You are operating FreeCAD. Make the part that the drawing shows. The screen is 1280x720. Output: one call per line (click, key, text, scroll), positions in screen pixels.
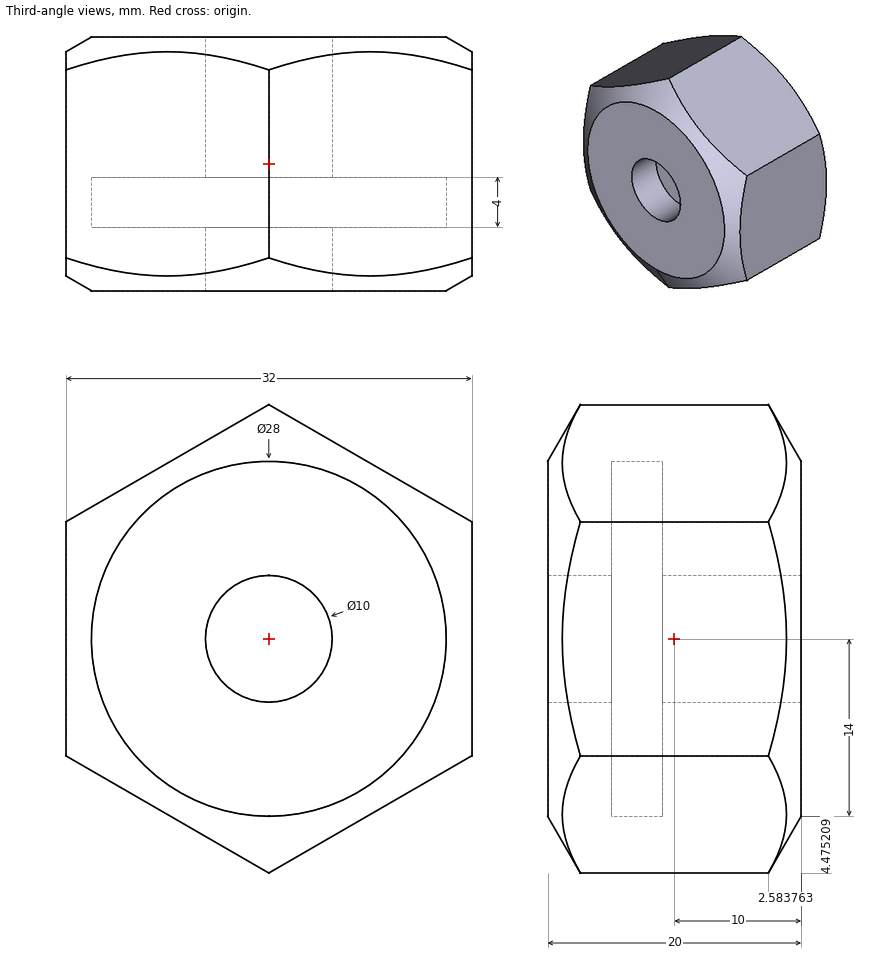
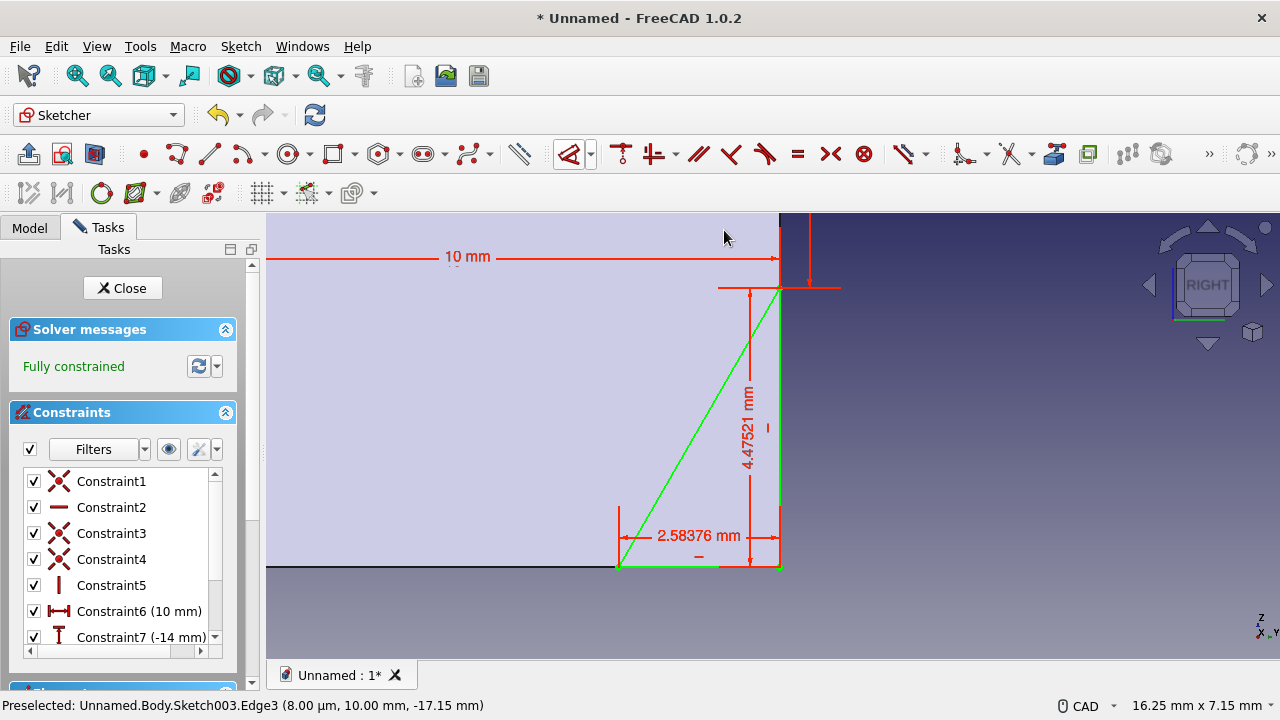
click(123, 288)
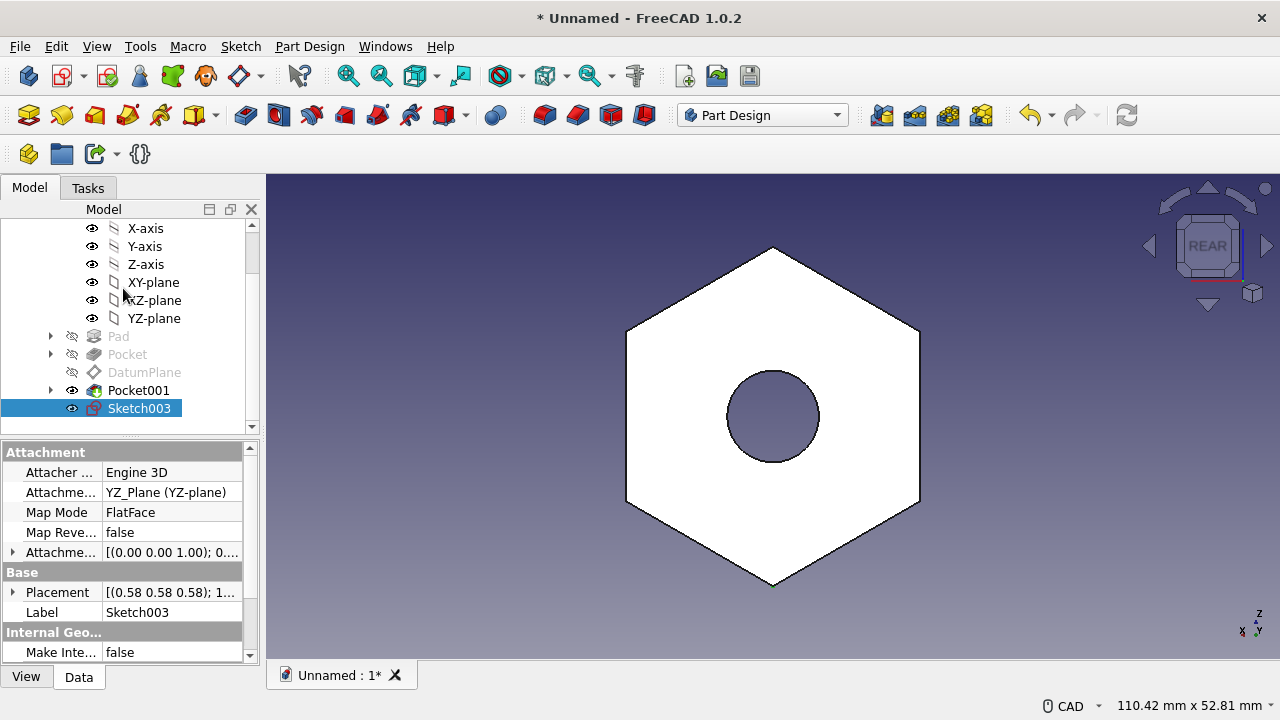
click(312, 116)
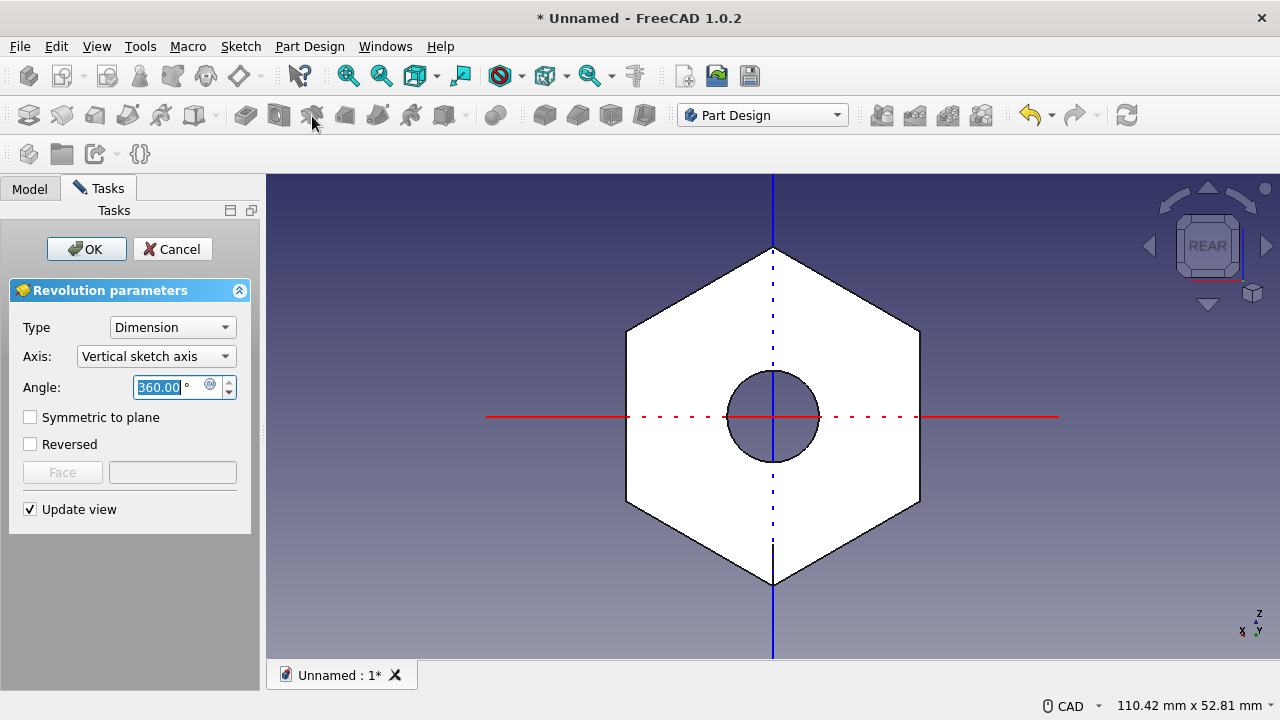
click(157, 356)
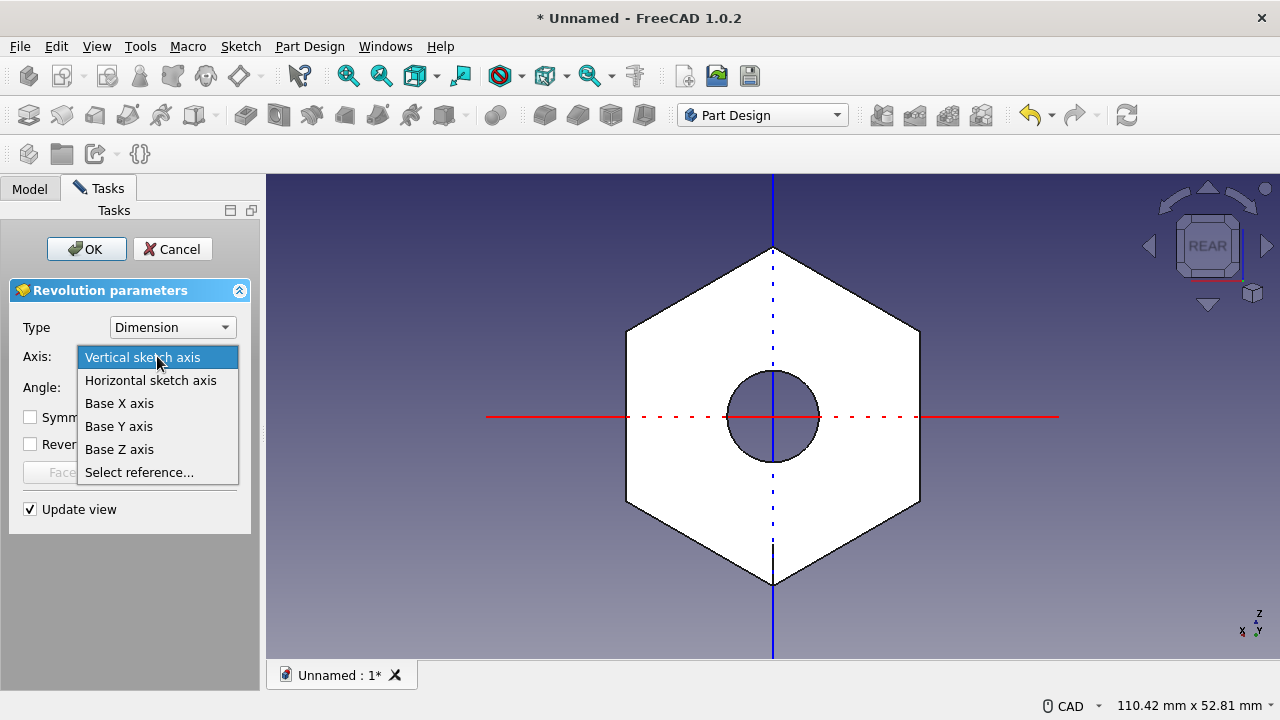
click(156, 380)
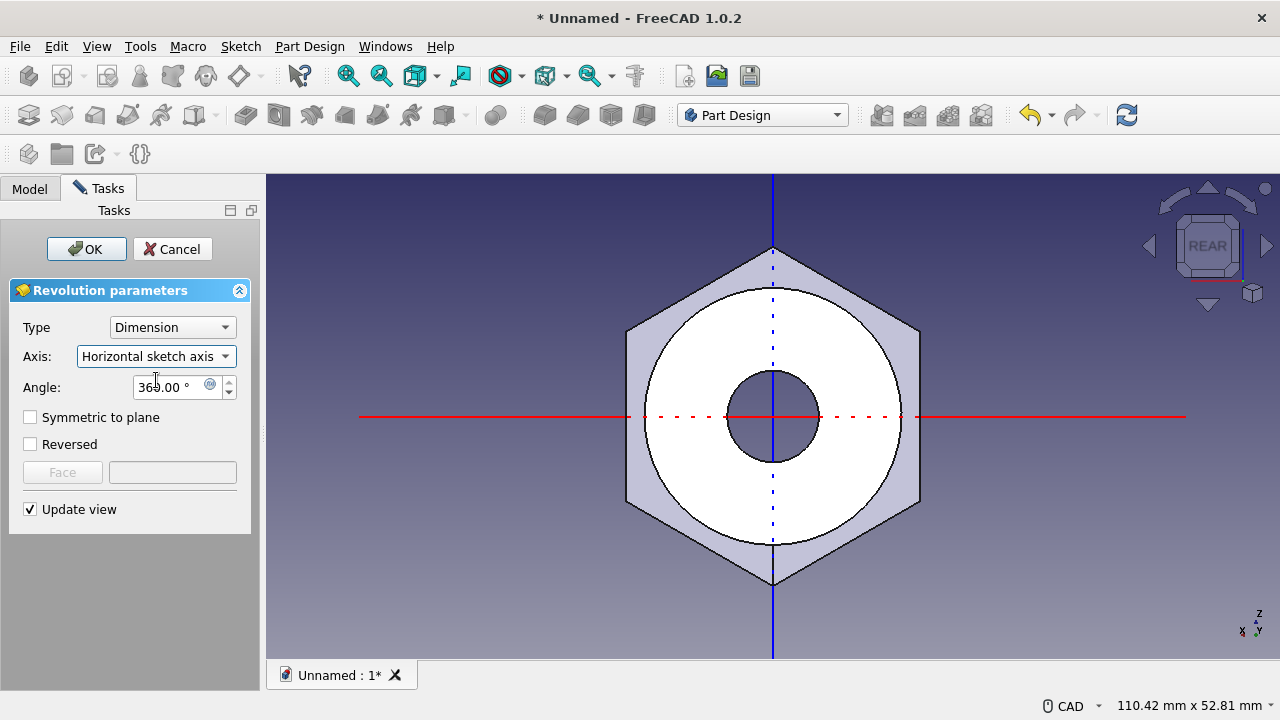
click(87, 249)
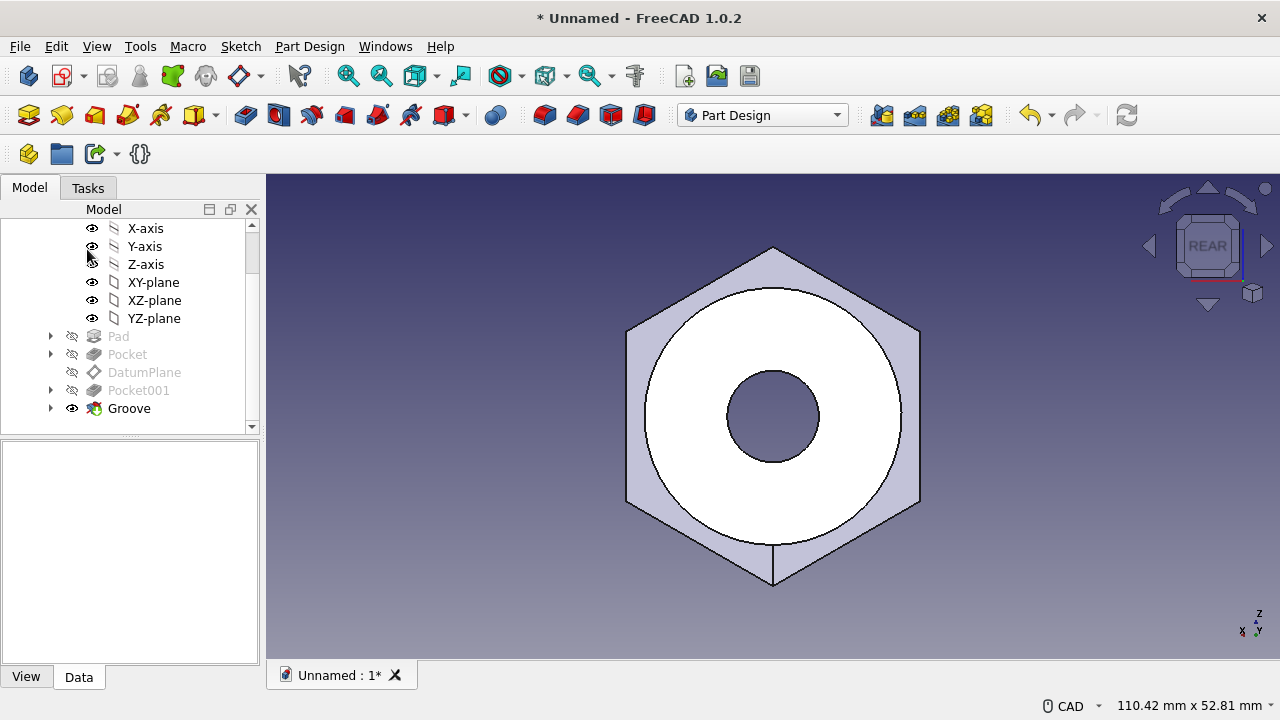
click(117, 408)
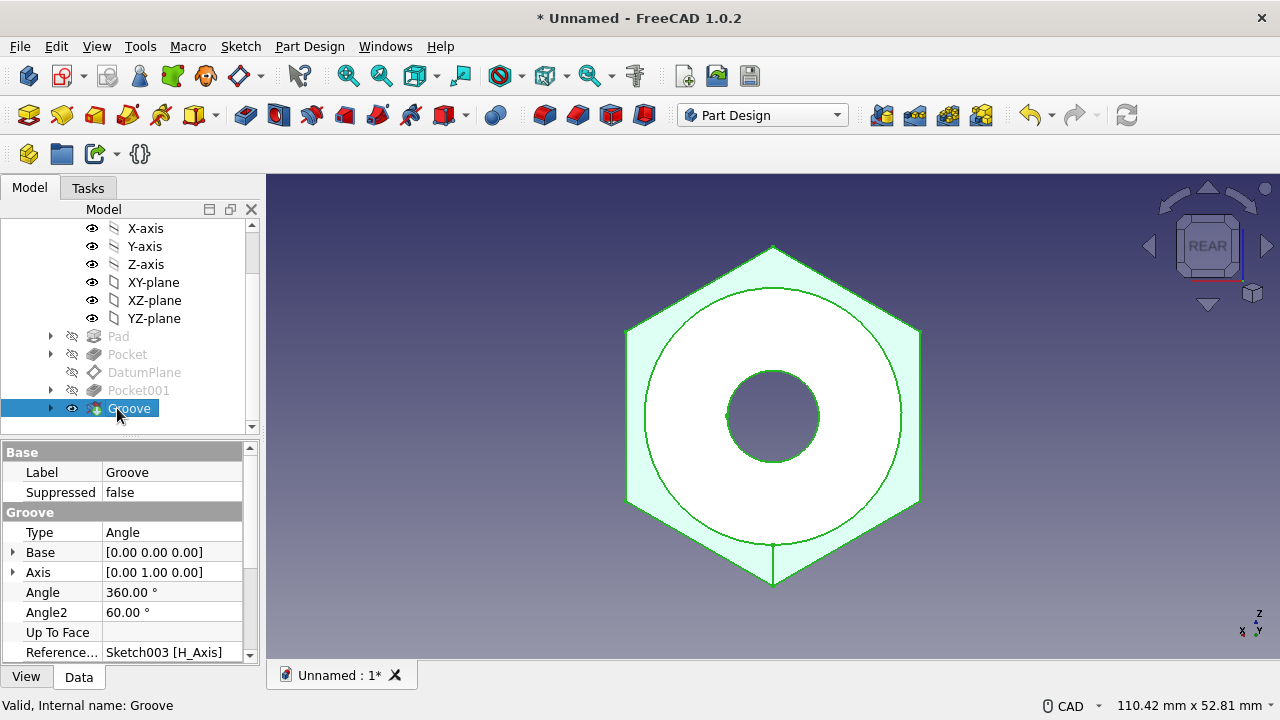
click(882, 116)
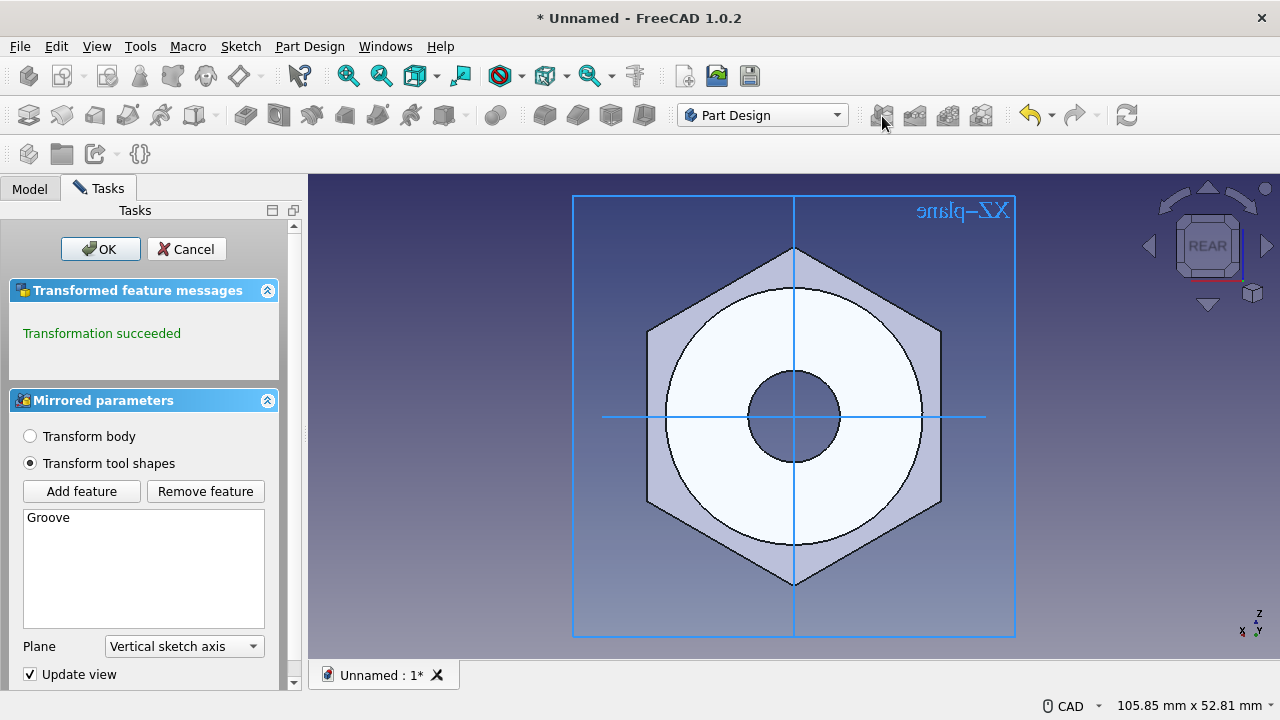
click(185, 646)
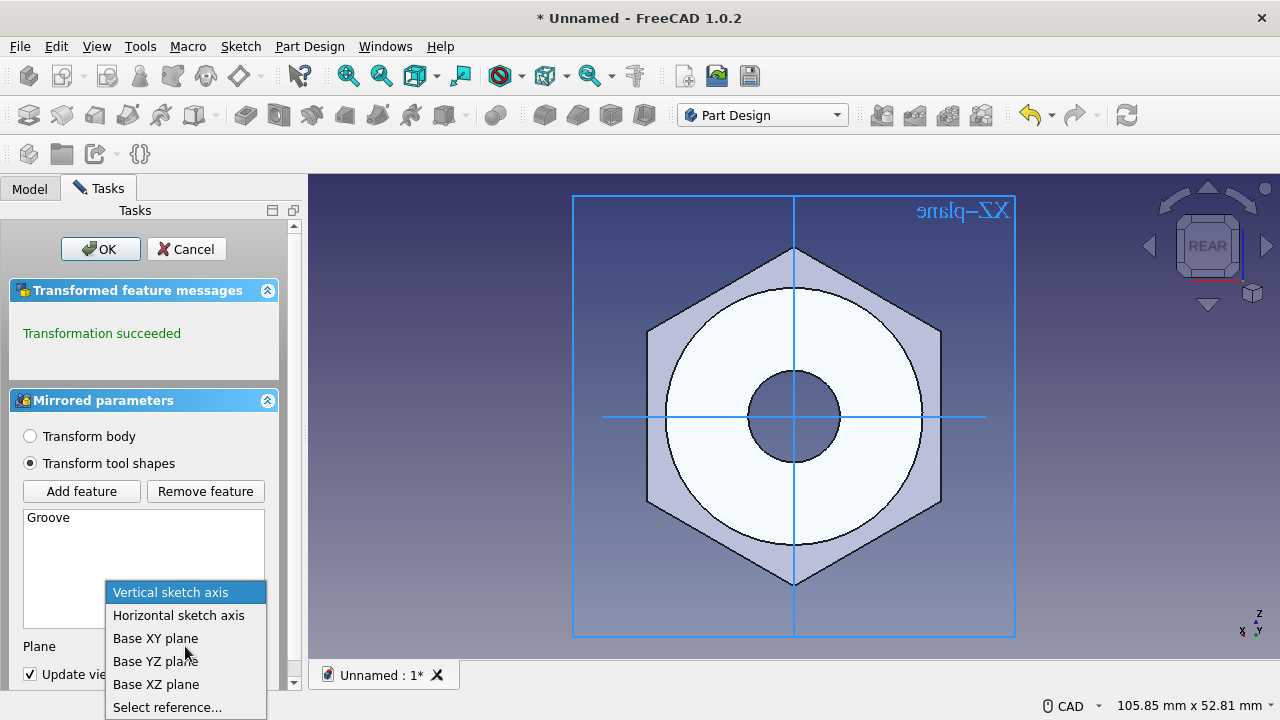
click(184, 684)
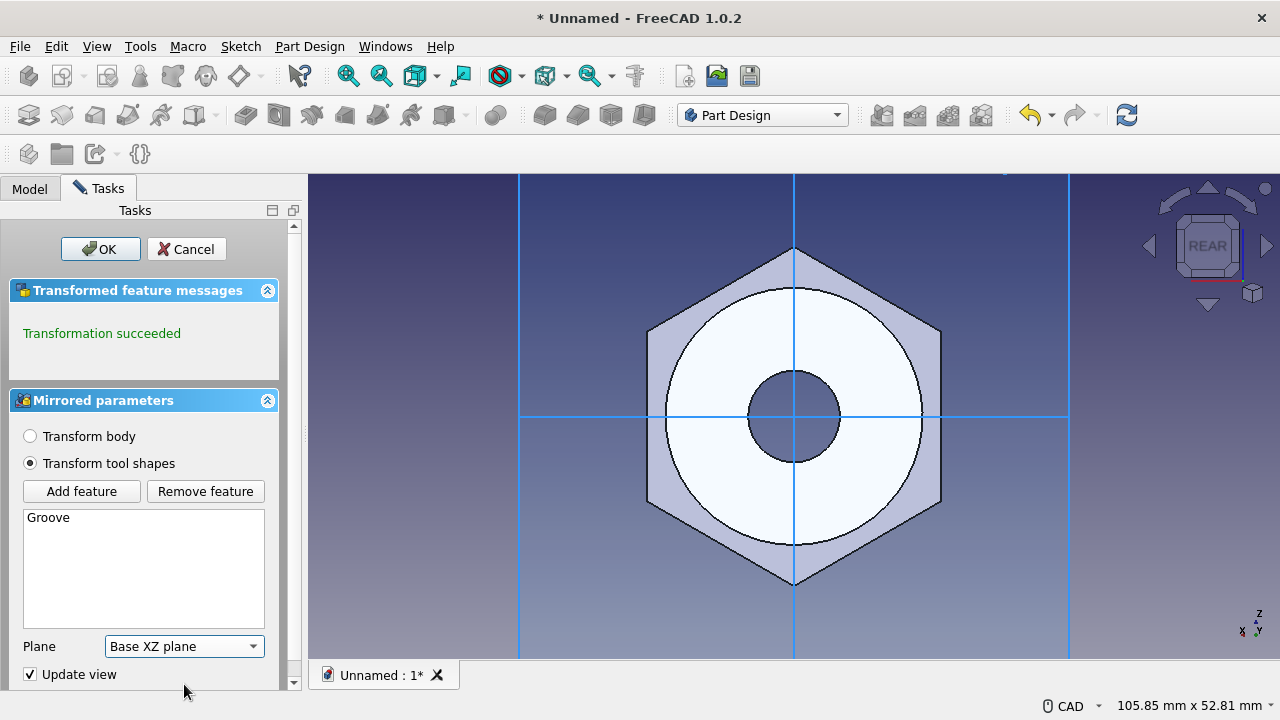
click(101, 249)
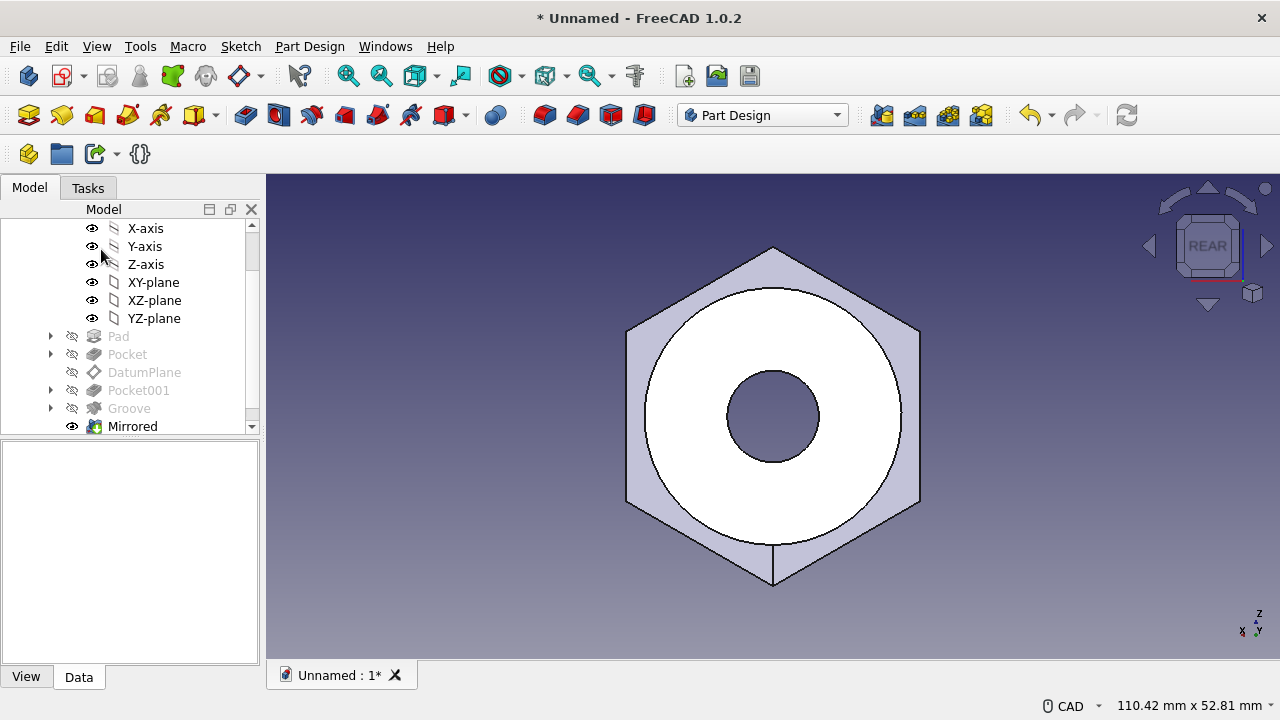
key(0)